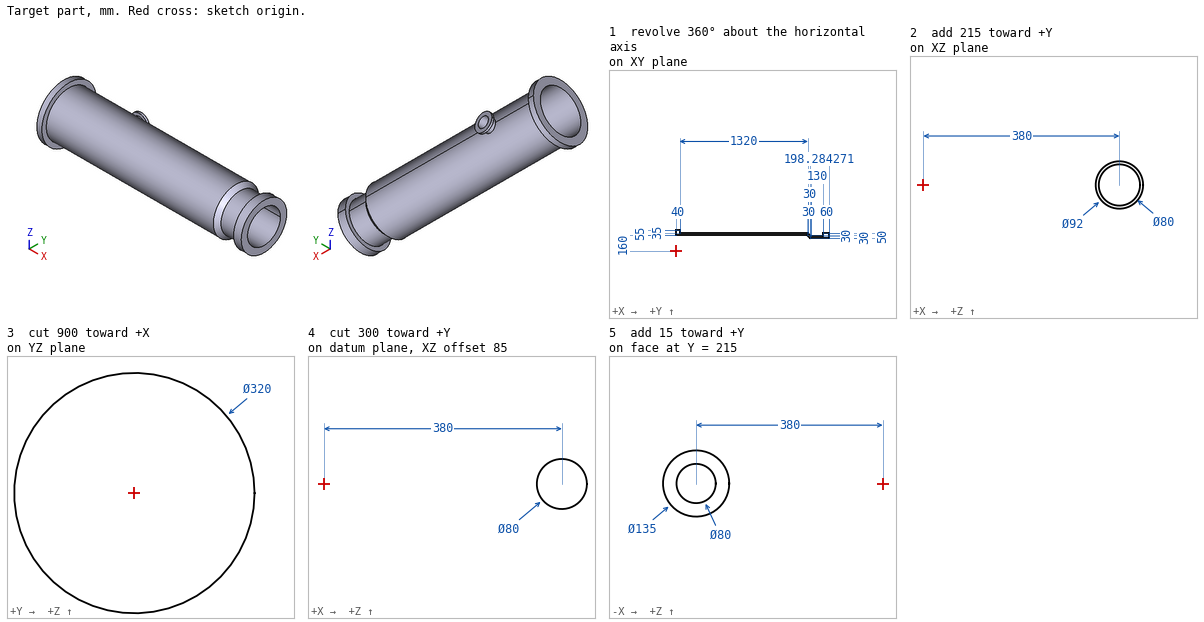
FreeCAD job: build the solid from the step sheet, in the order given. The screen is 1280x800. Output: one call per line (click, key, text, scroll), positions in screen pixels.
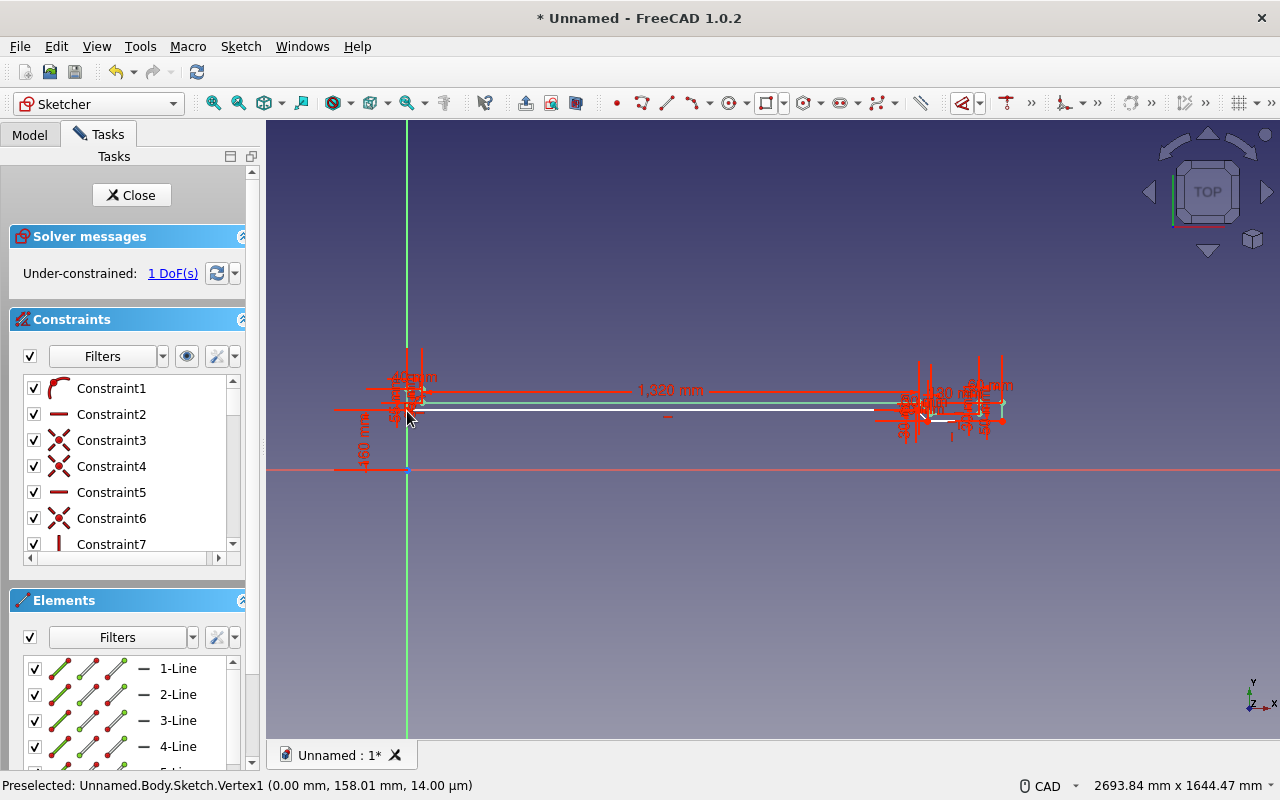
scroll(987, 421, up, 2)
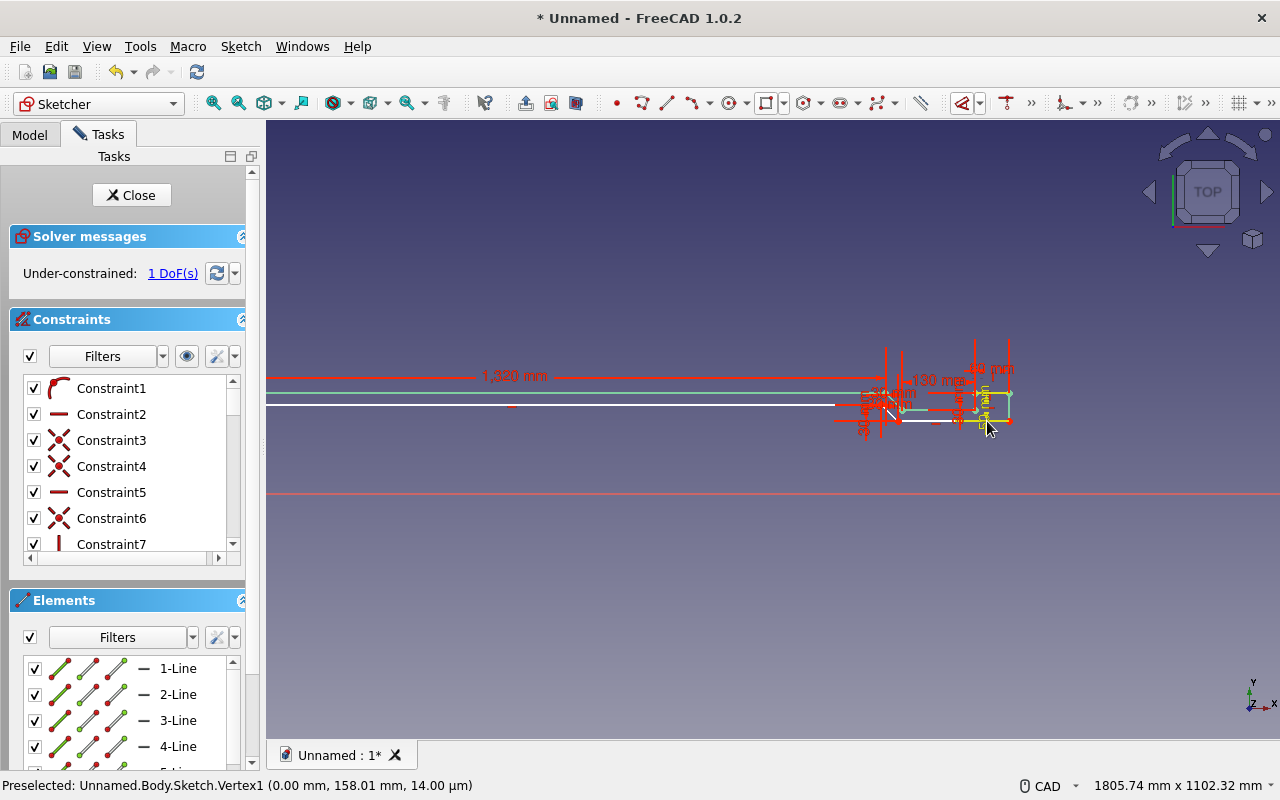
click(976, 421)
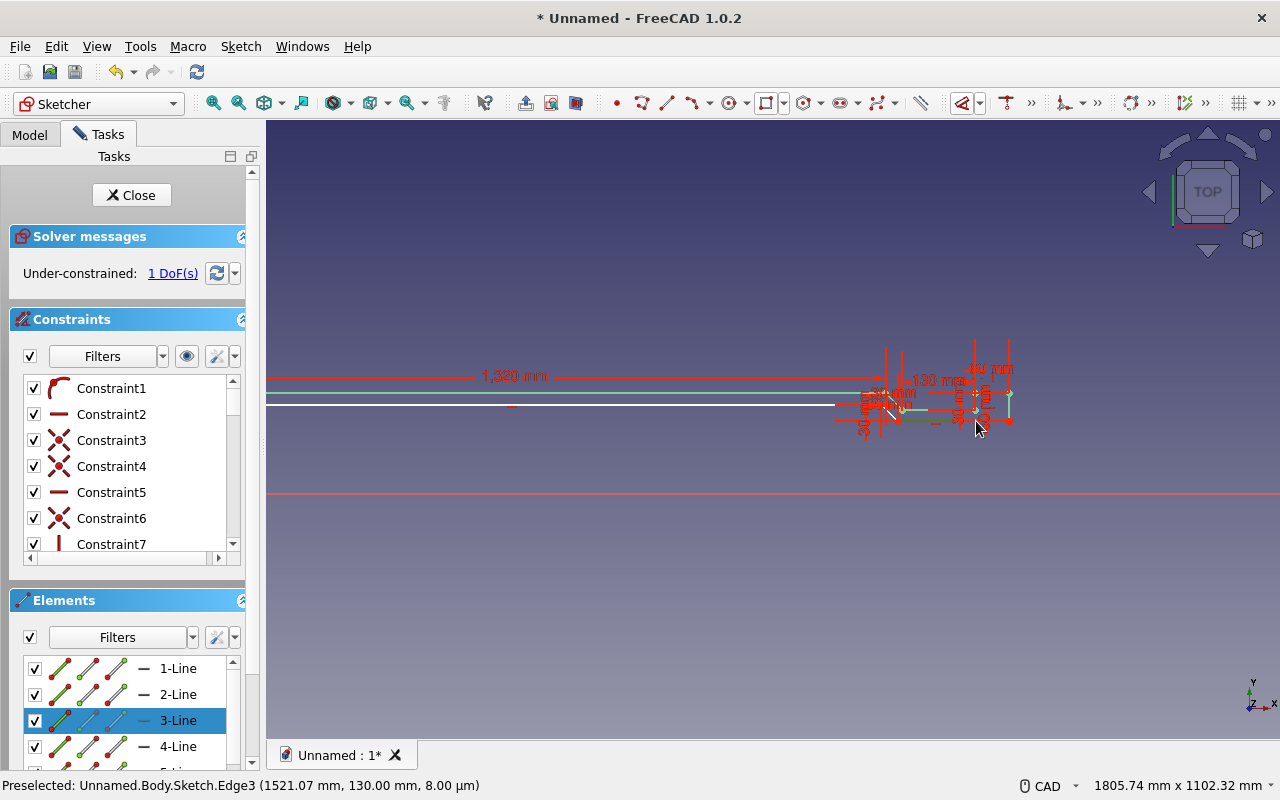
key(l)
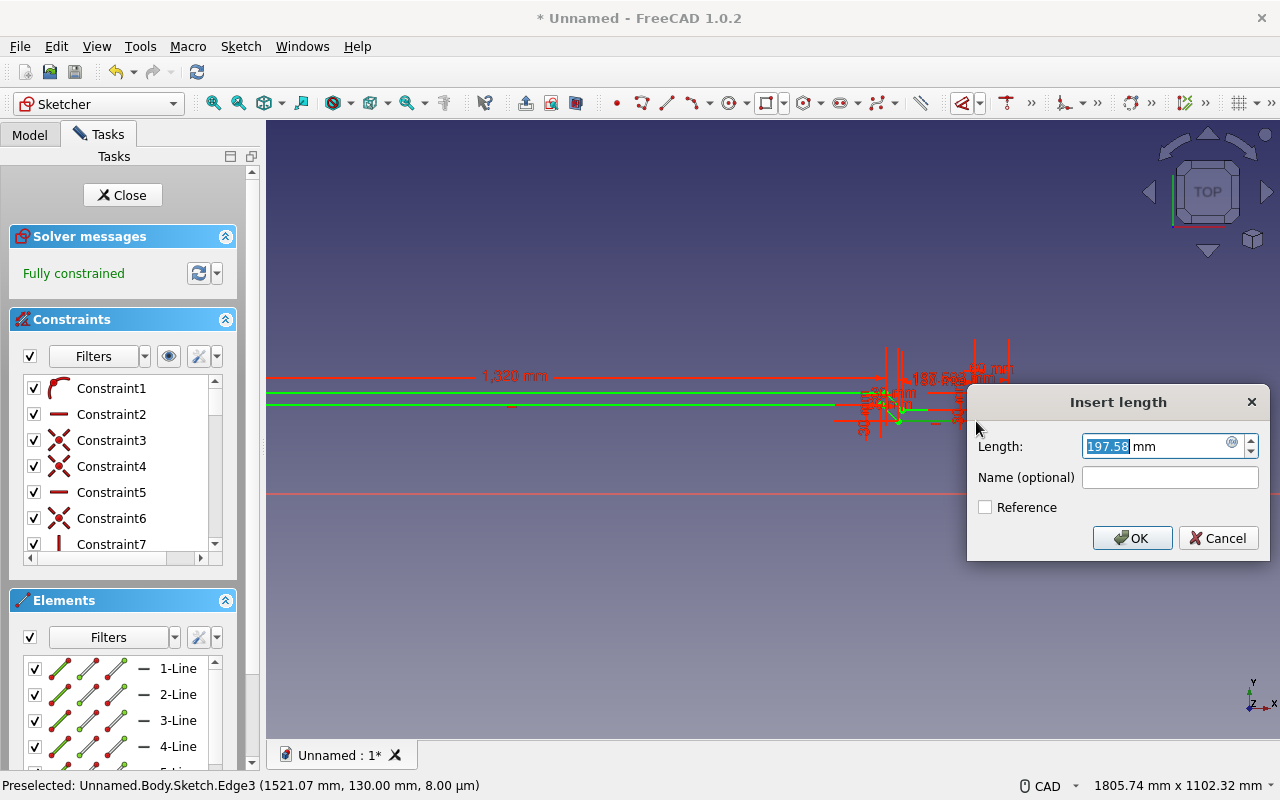
text(198.284271)
key(Return)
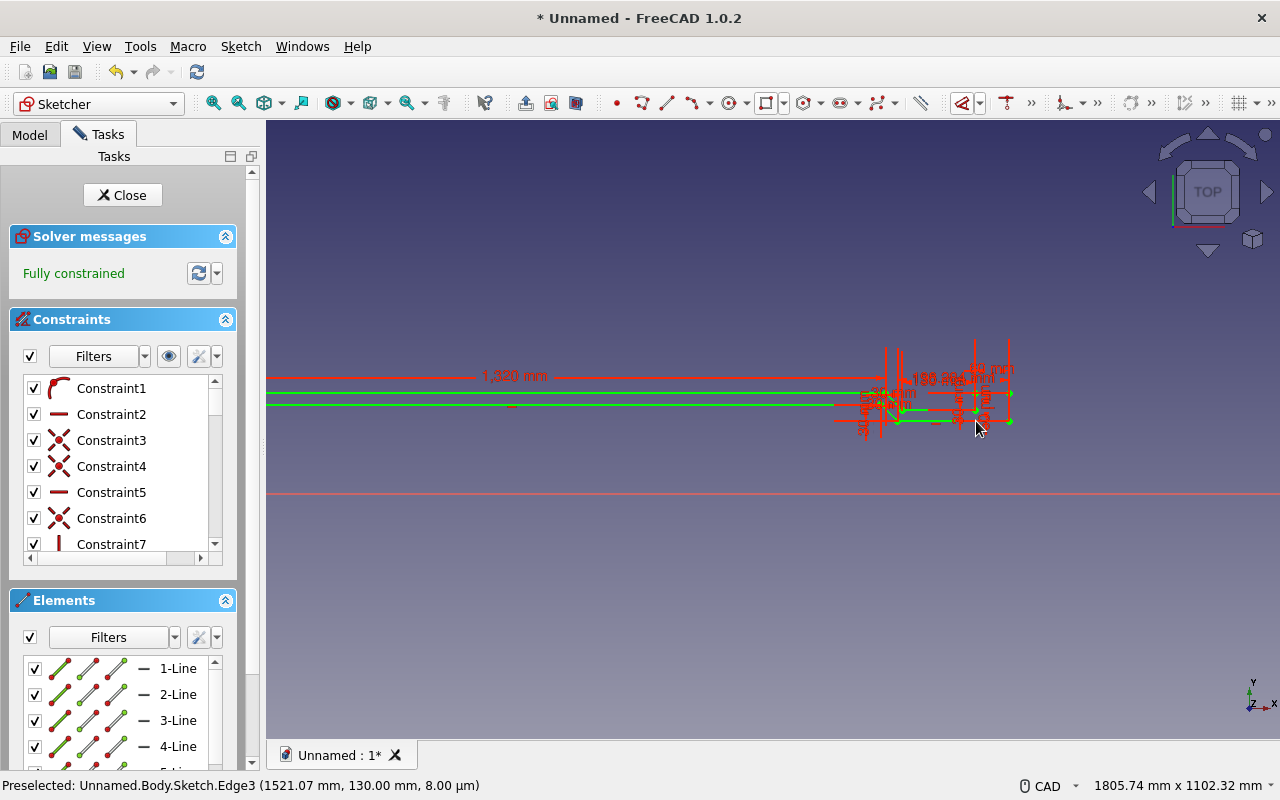
click(123, 195)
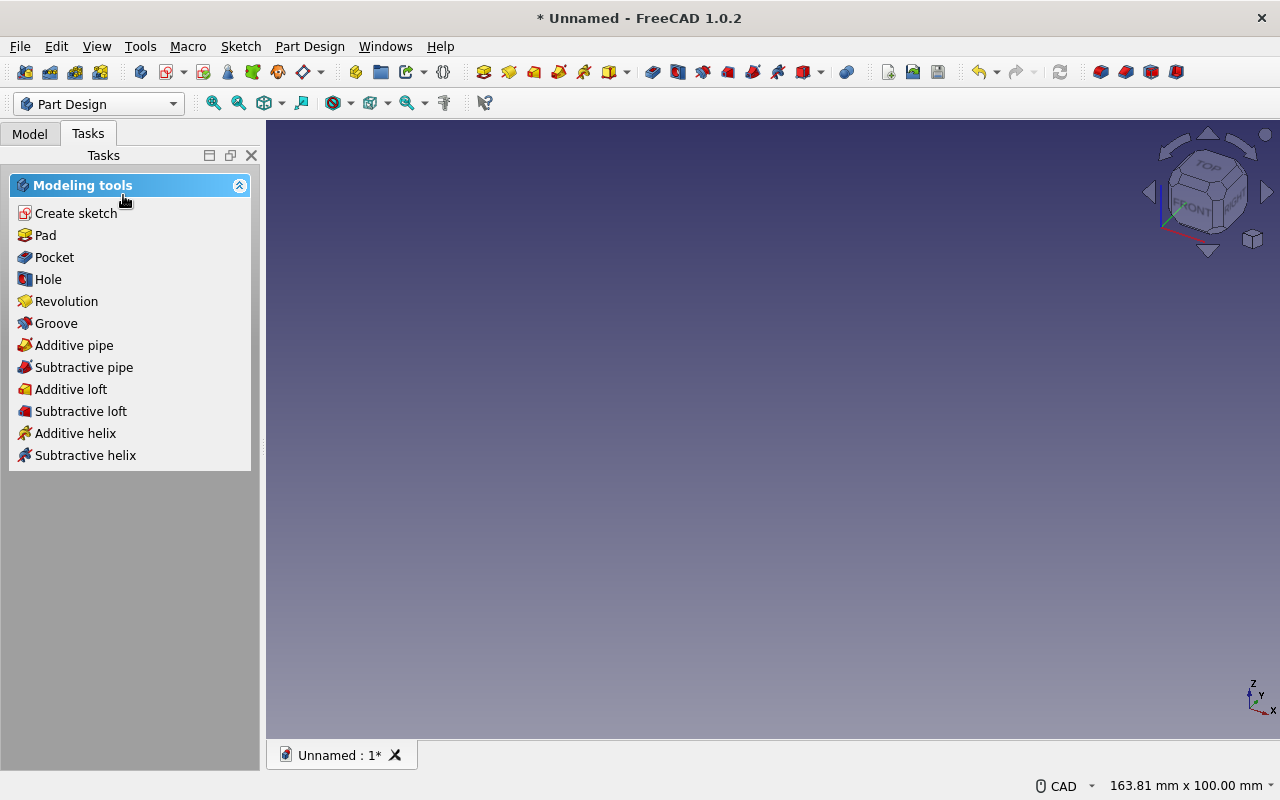
click(509, 72)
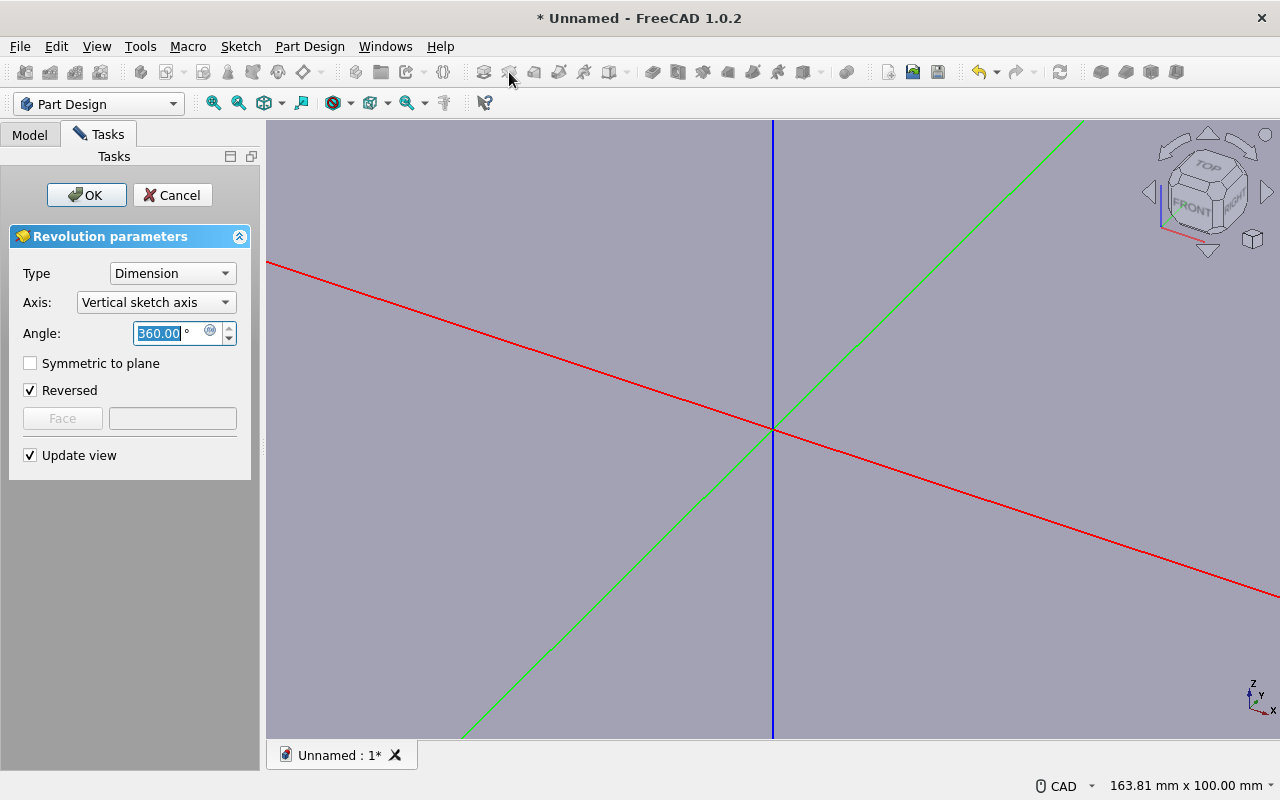
click(157, 302)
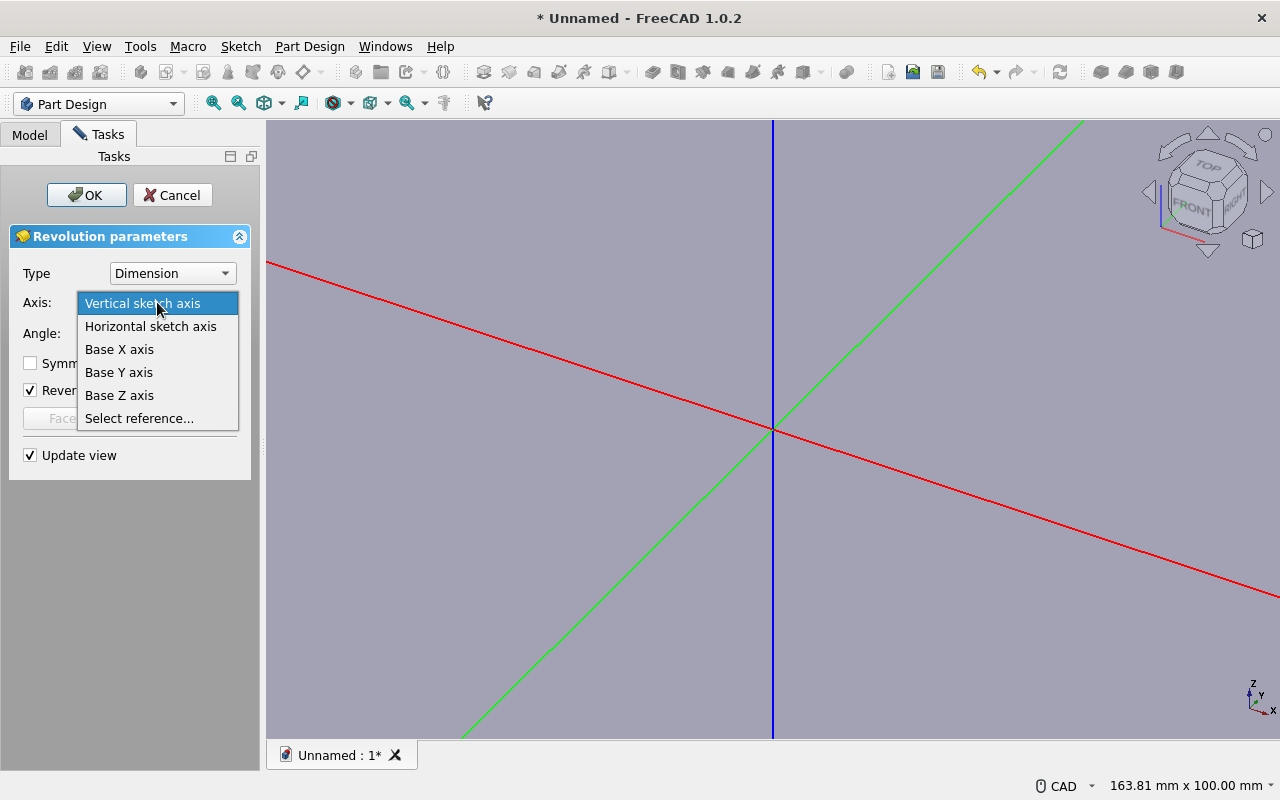
click(156, 326)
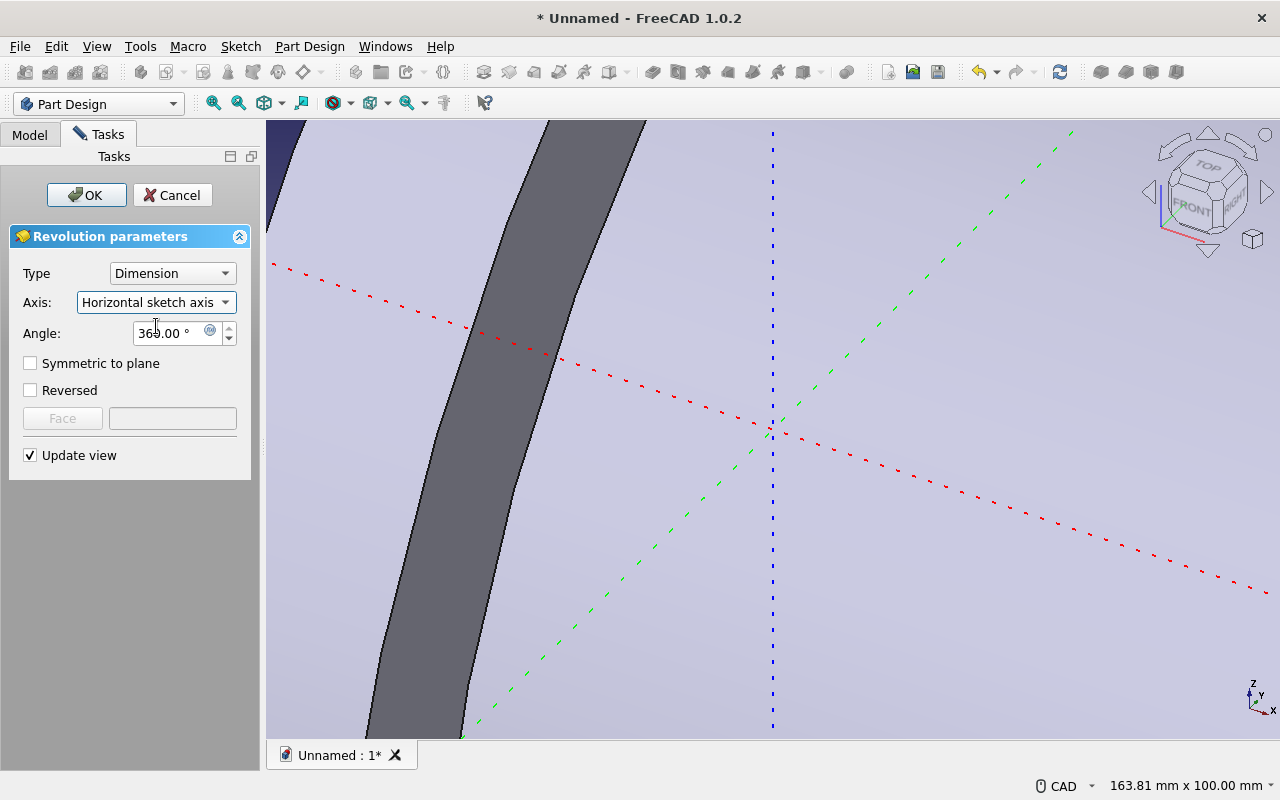
click(87, 195)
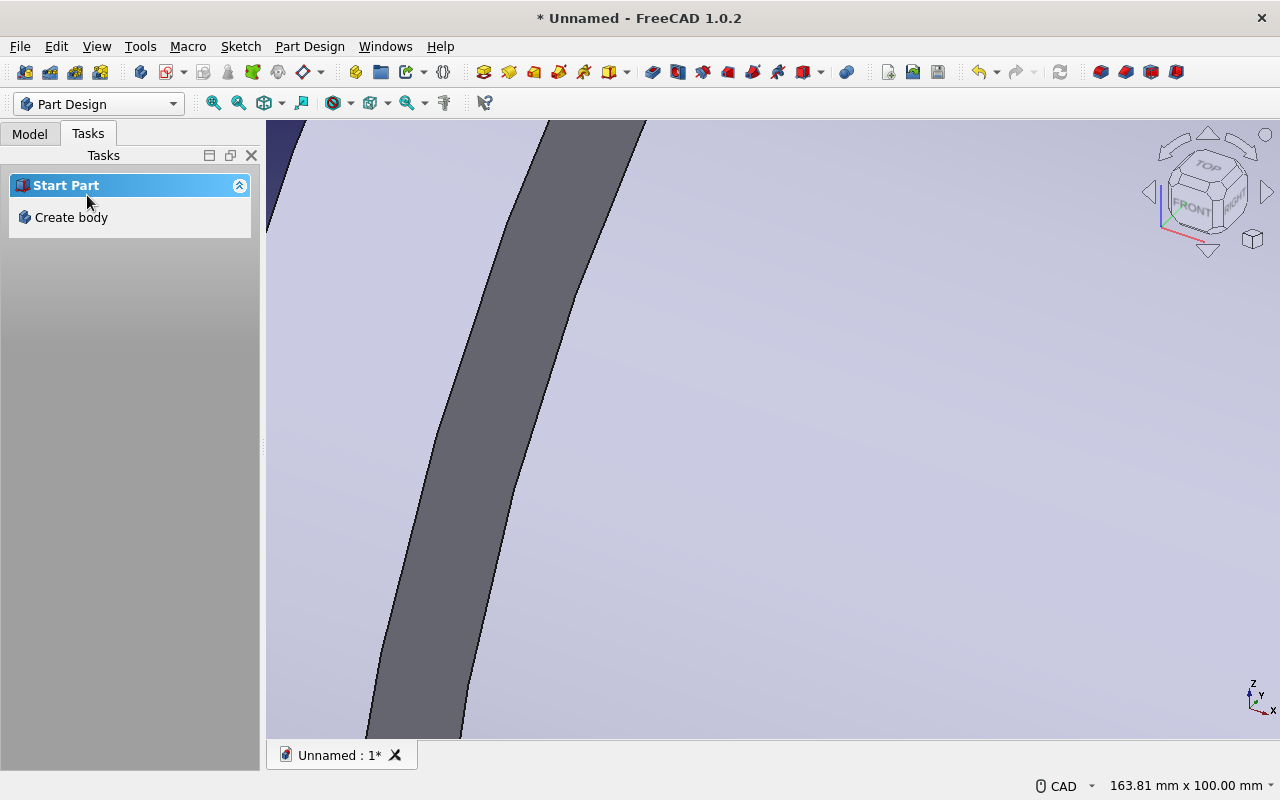
key(v)
key(f)